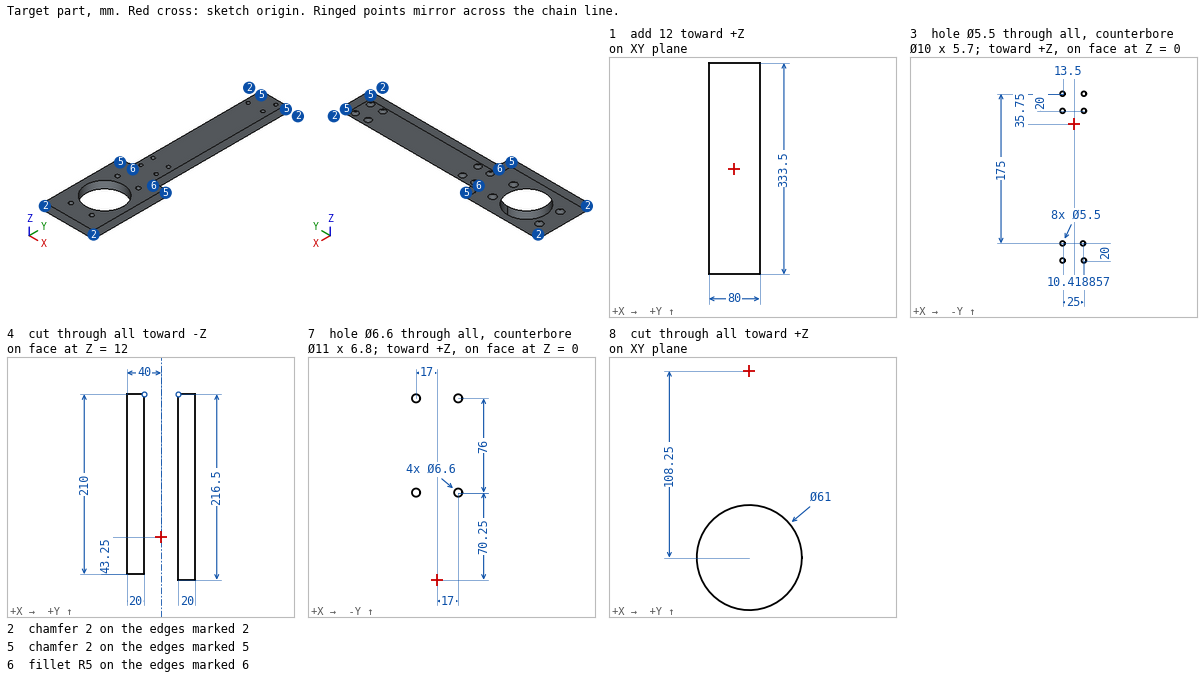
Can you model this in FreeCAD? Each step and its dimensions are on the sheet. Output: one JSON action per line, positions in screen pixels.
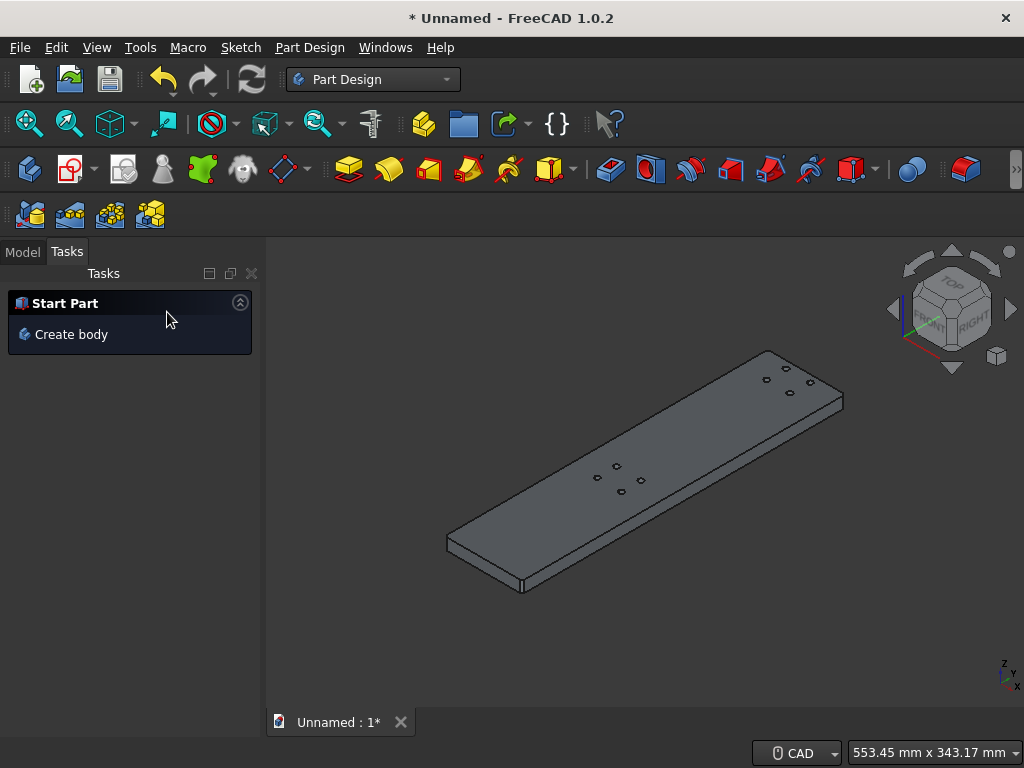
{"action": "left_click", "coordinate": [737, 411]}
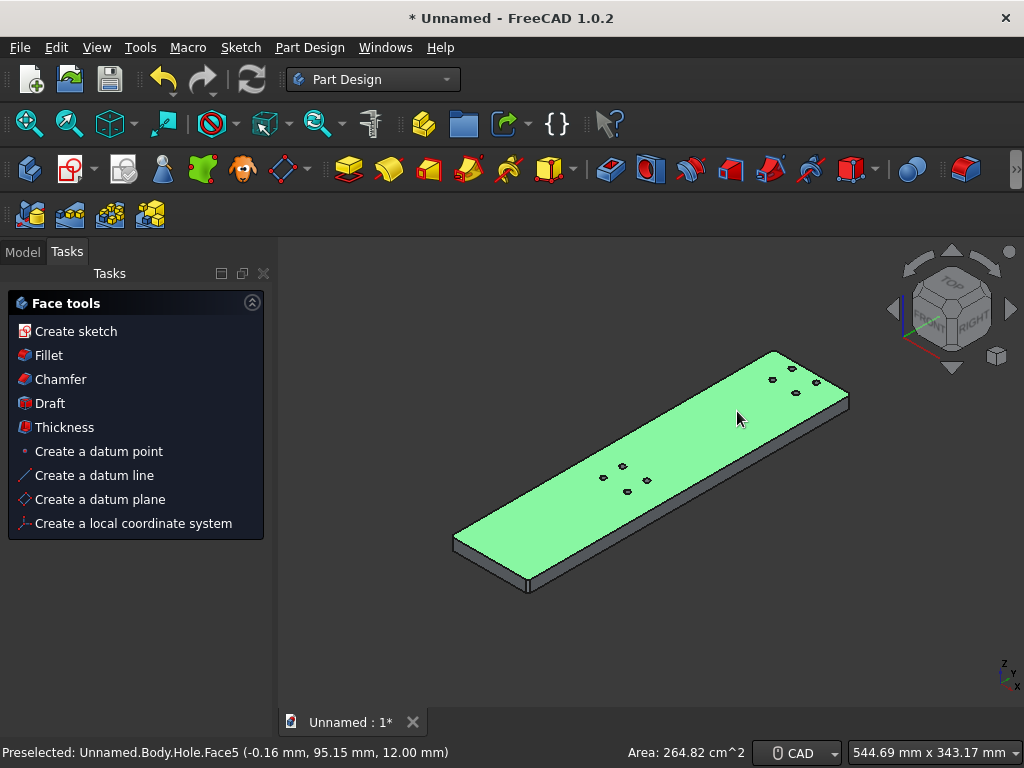
{"action": "left_click", "coordinate": [70, 170]}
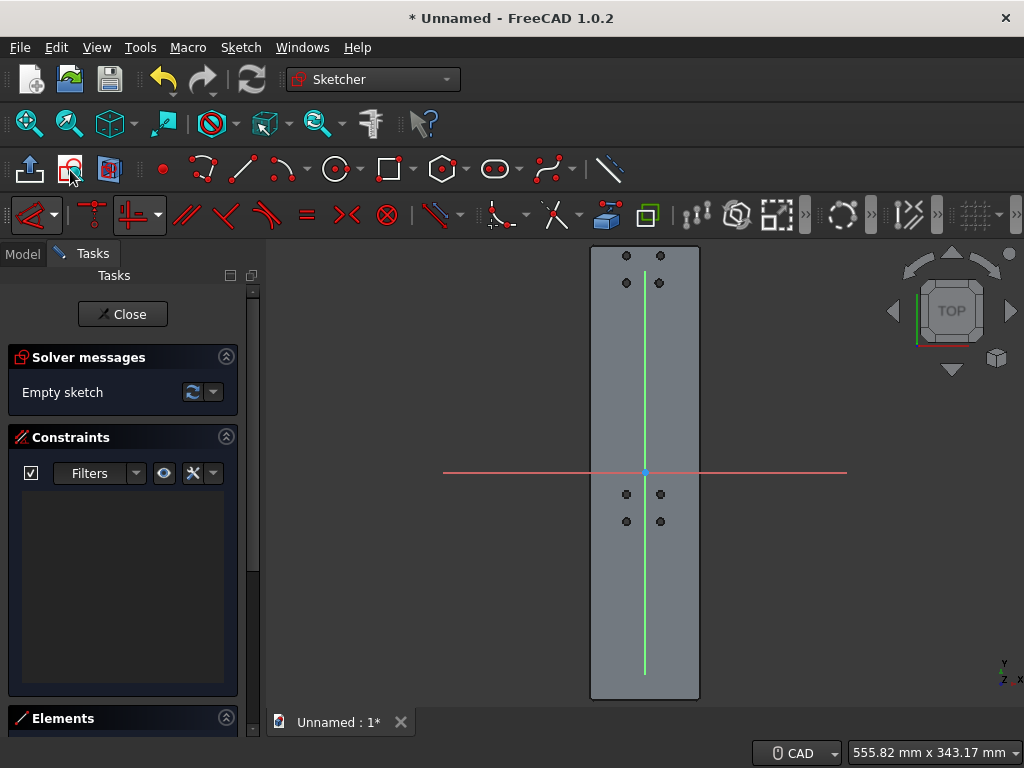
{"action": "scroll", "coordinate": [294, 679], "scroll_direction": "down", "scroll_amount": 1}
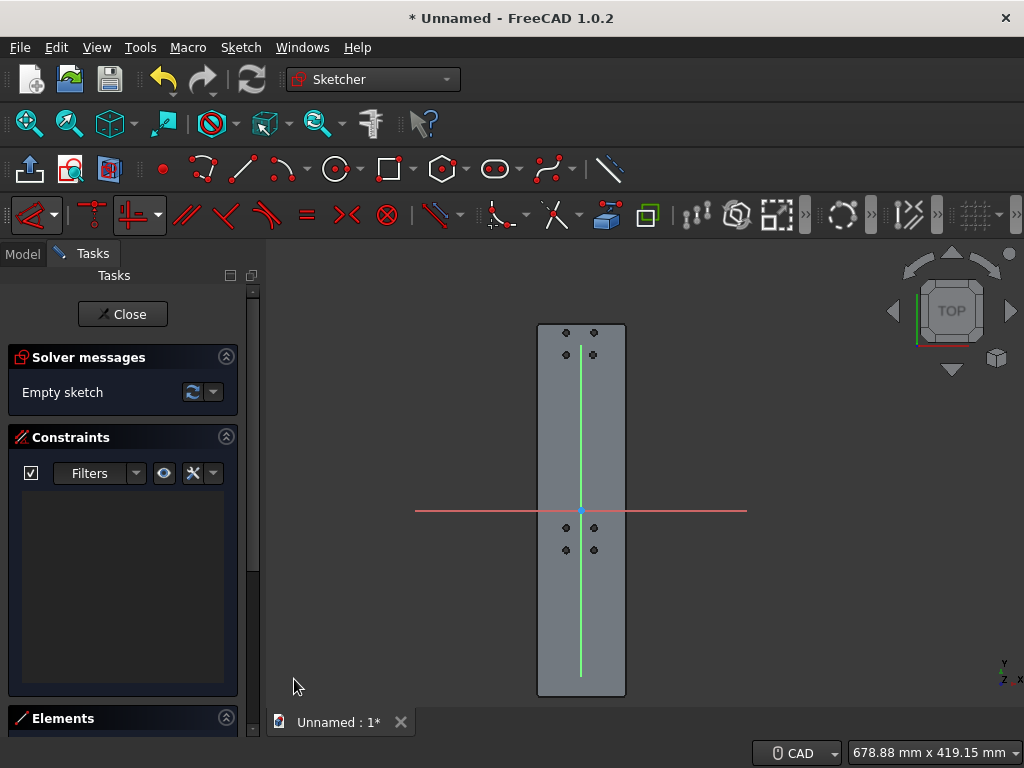
{"action": "key", "text": "g r"}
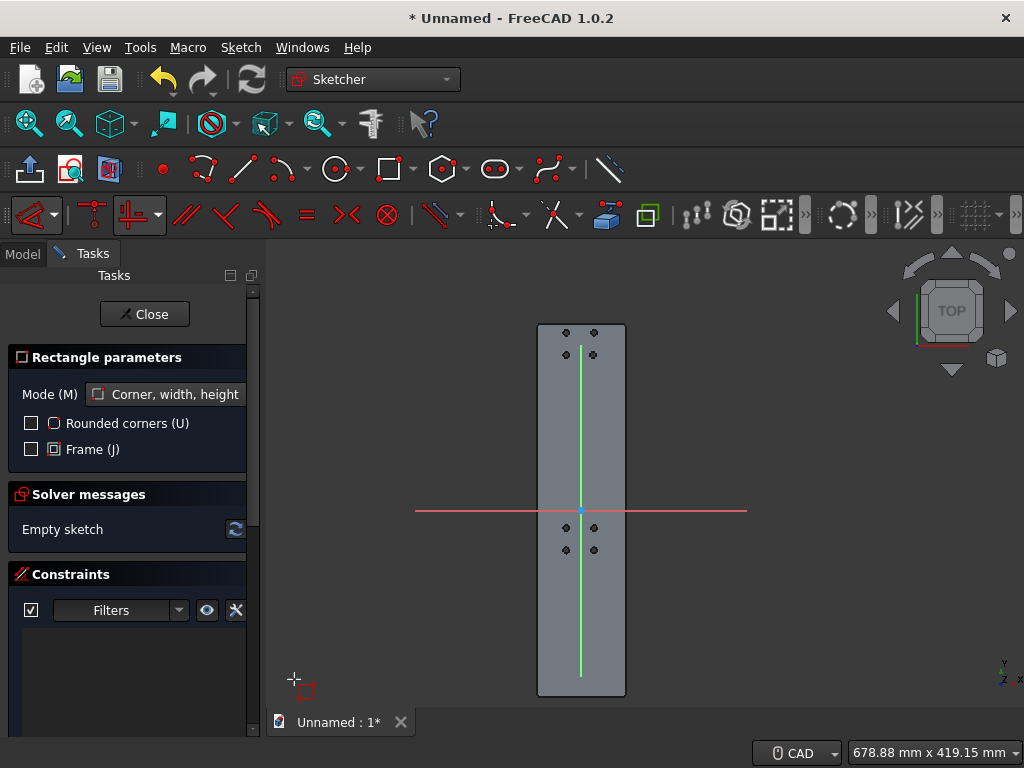
{"action": "left_click", "coordinate": [537, 324]}
{"action": "left_click", "coordinate": [559, 559]}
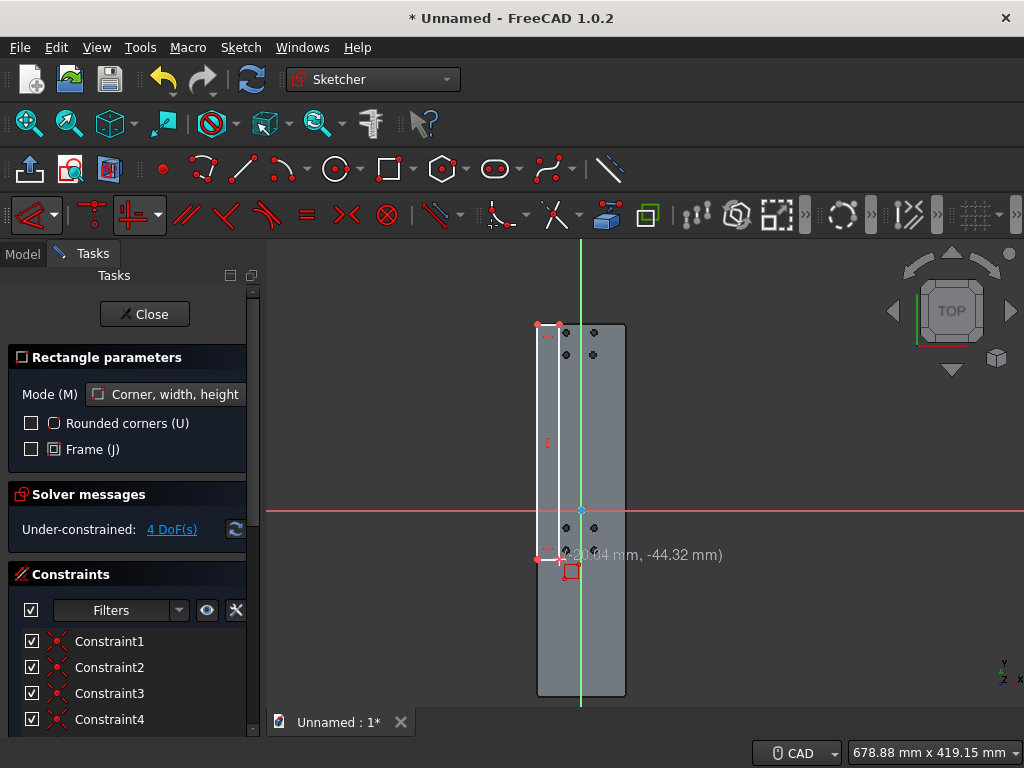
{"action": "left_click", "coordinate": [604, 324]}
{"action": "left_click", "coordinate": [626, 566]}
{"action": "key", "text": "Escape"}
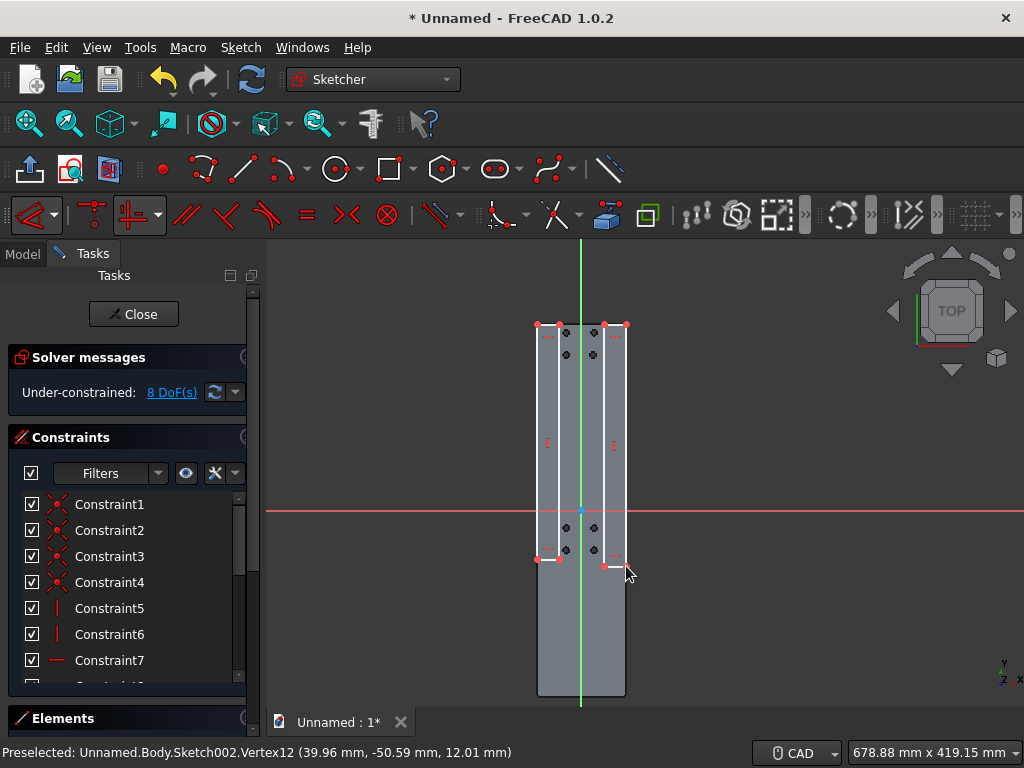
{"action": "left_click", "coordinate": [559, 325]}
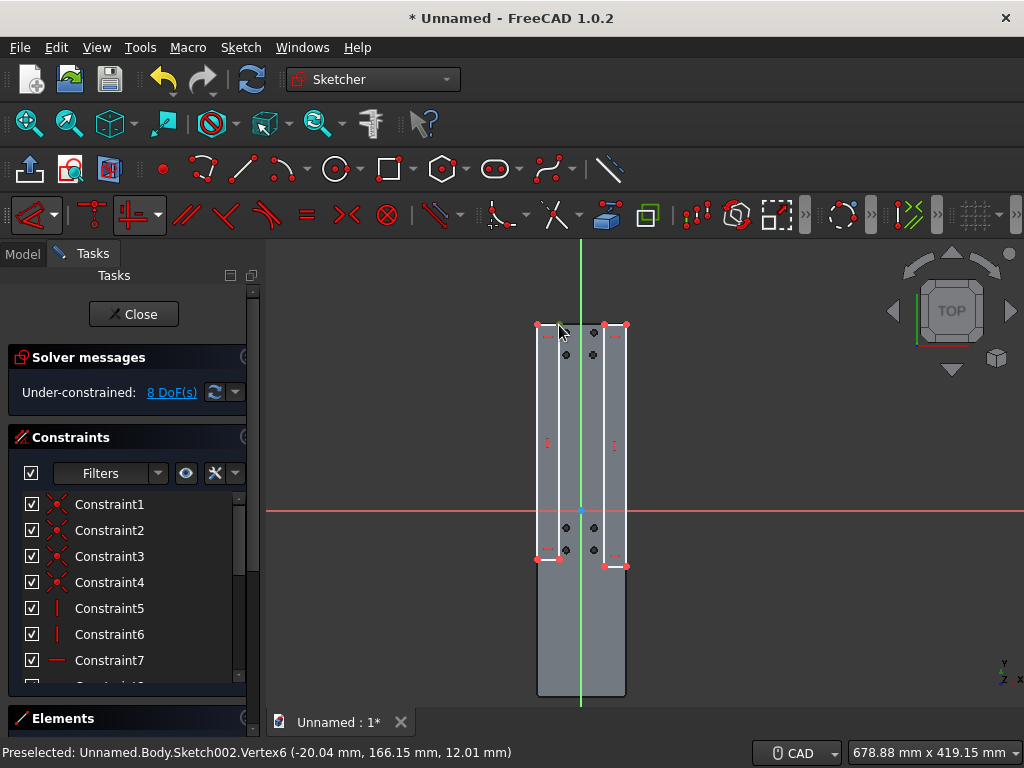
{"action": "left_click", "coordinate": [604, 325]}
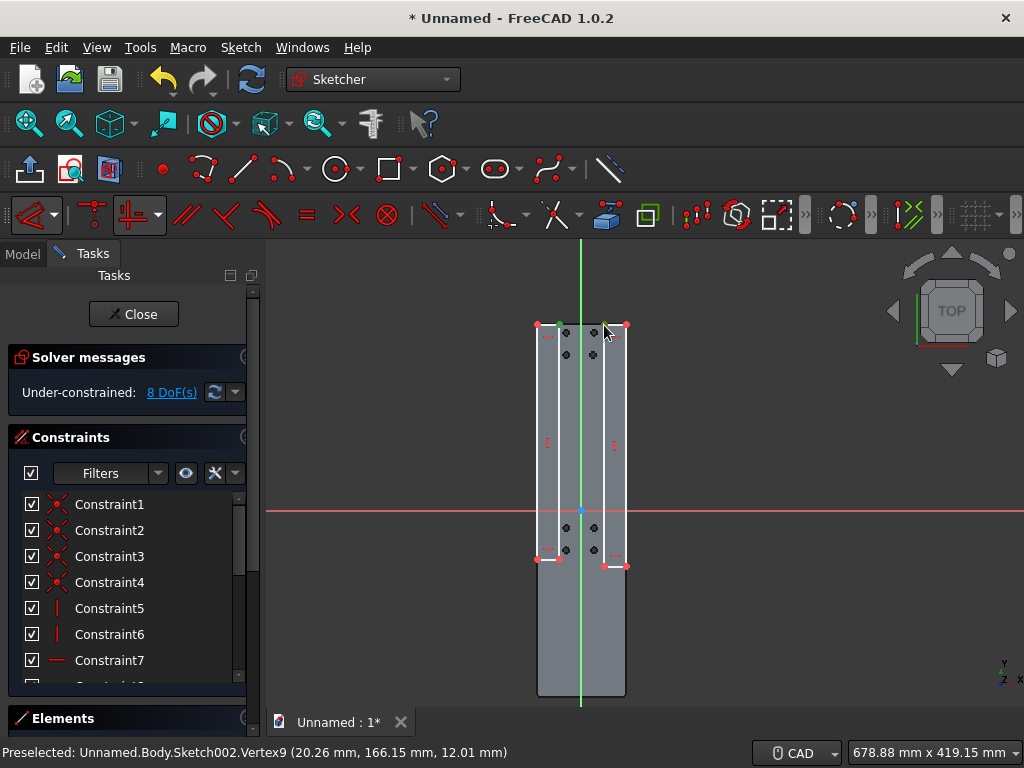
{"action": "left_click", "coordinate": [581, 650]}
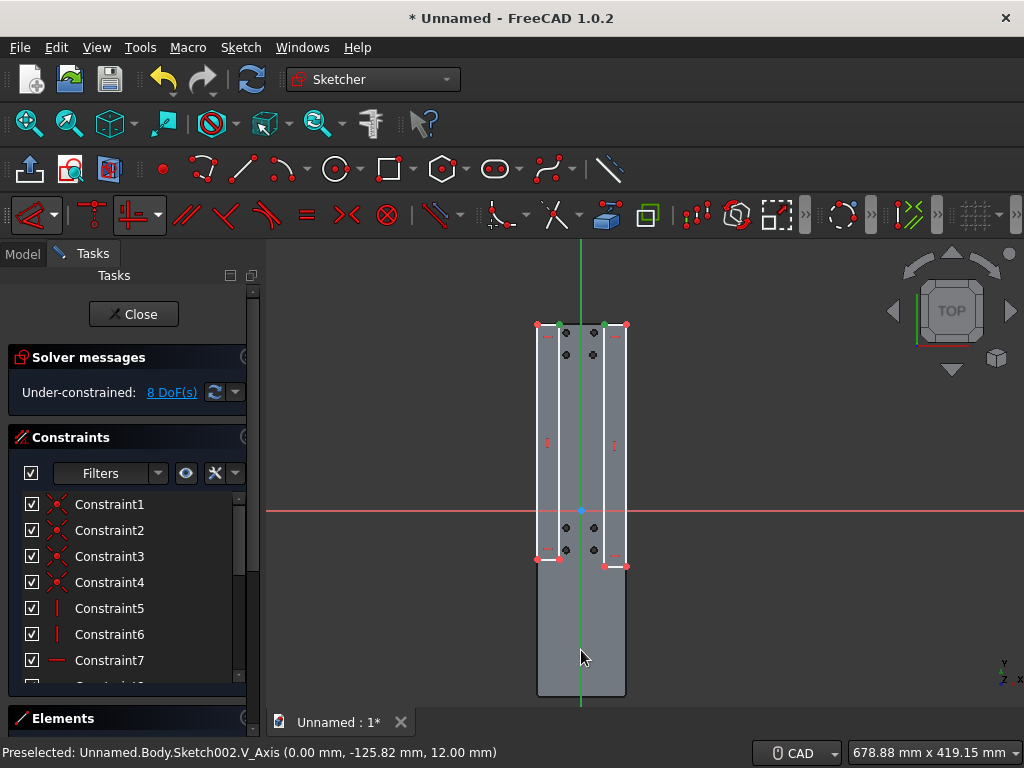
{"action": "left_click", "coordinate": [348, 216]}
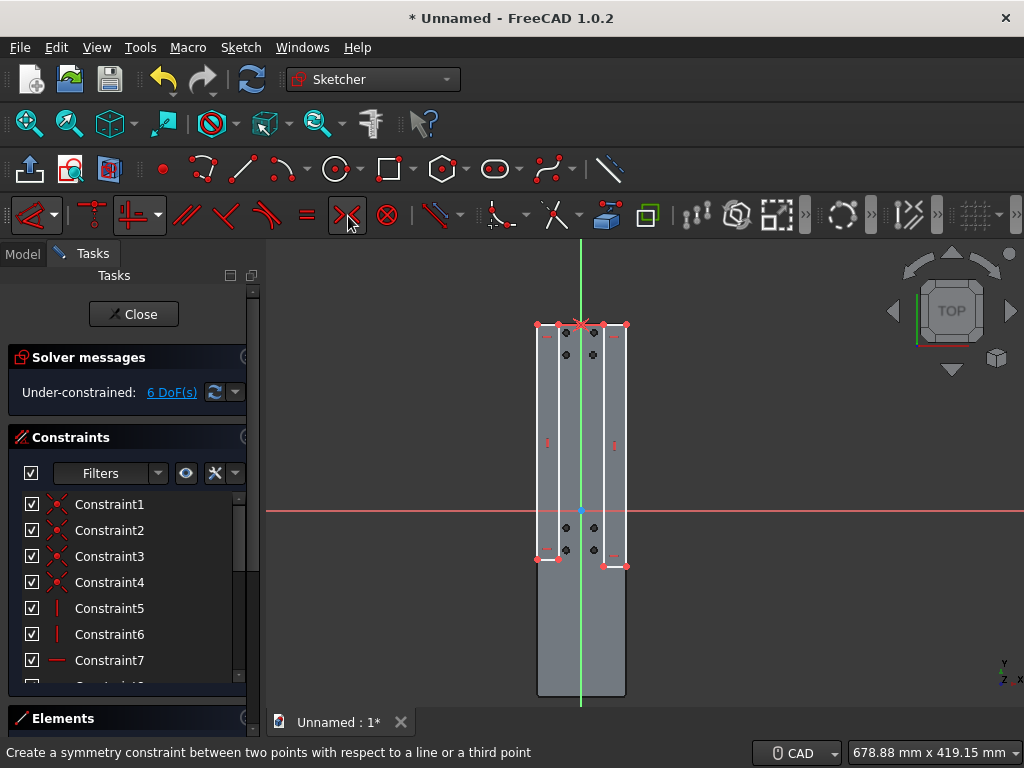
{"action": "left_click", "coordinate": [30, 216]}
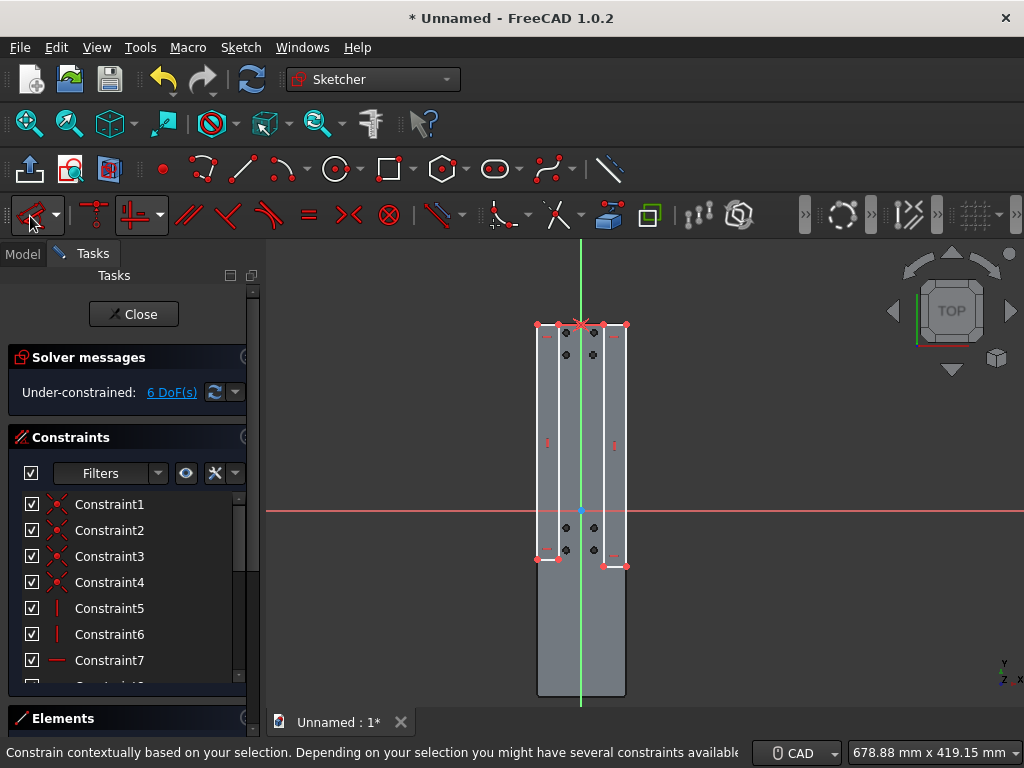
{"action": "scroll", "coordinate": [548, 560], "scroll_direction": "up", "scroll_amount": 3}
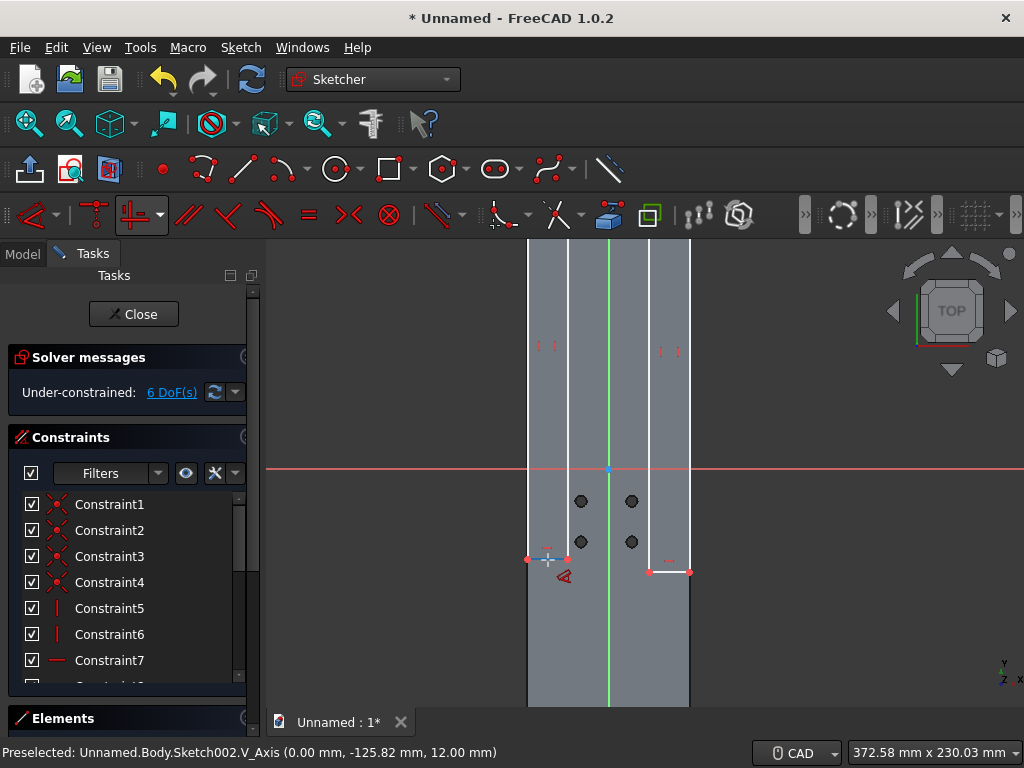
{"action": "left_click", "coordinate": [548, 559]}
{"action": "left_click", "coordinate": [548, 593]}